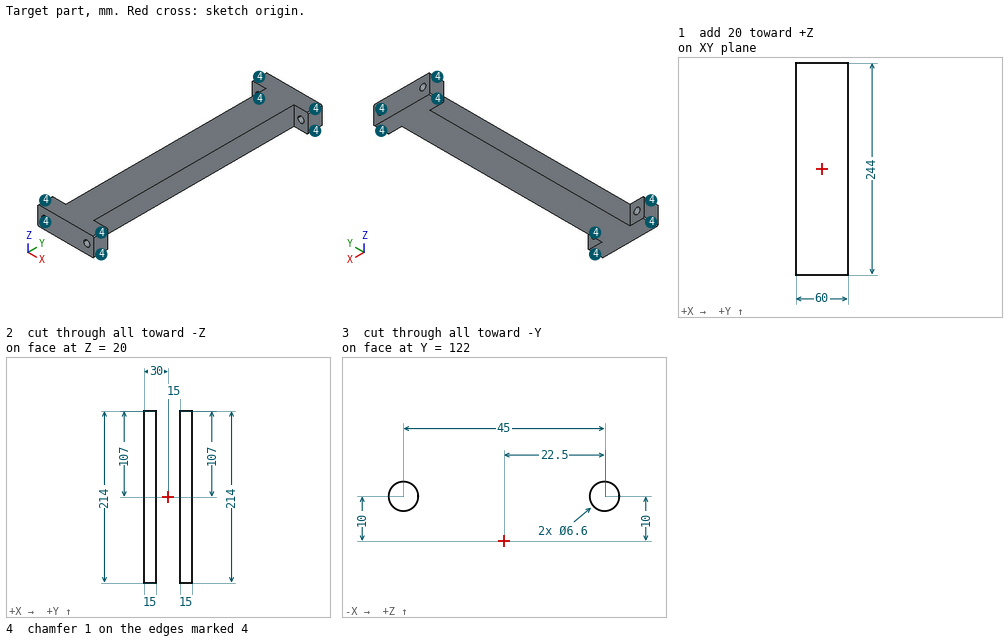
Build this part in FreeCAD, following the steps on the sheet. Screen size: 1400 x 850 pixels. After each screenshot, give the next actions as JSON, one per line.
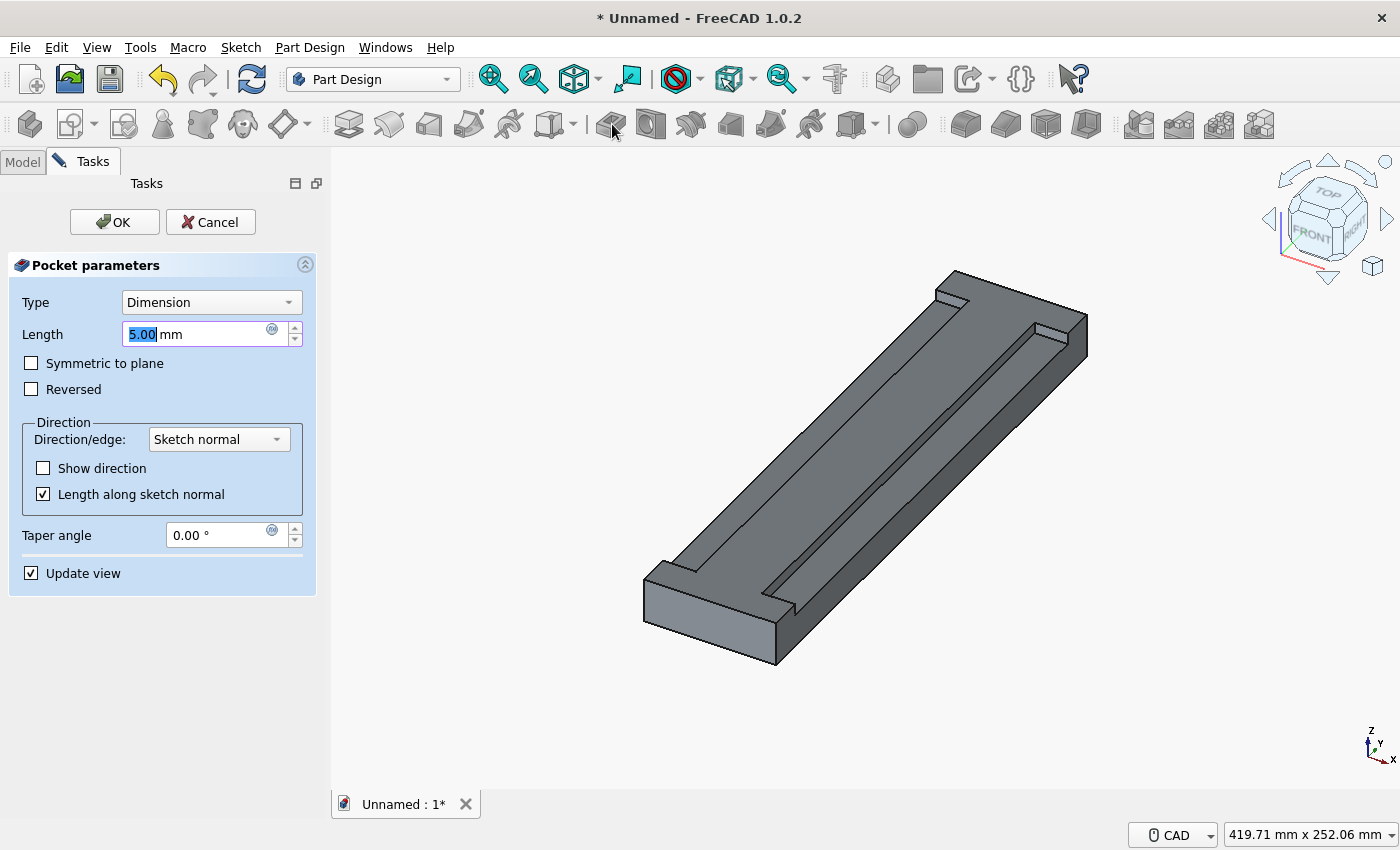
{"action": "left_click", "coordinate": [212, 302]}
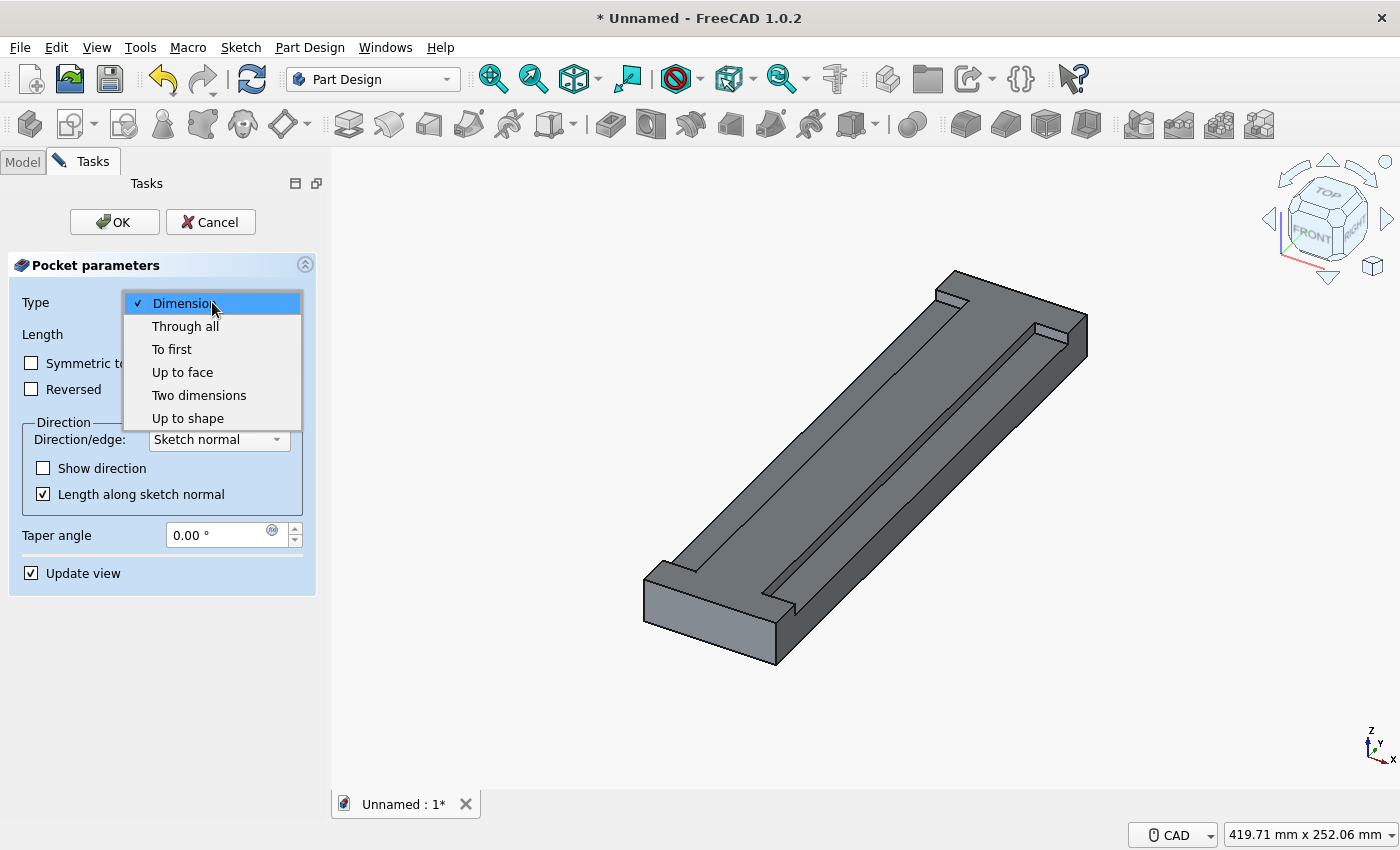
{"action": "left_click", "coordinate": [212, 326]}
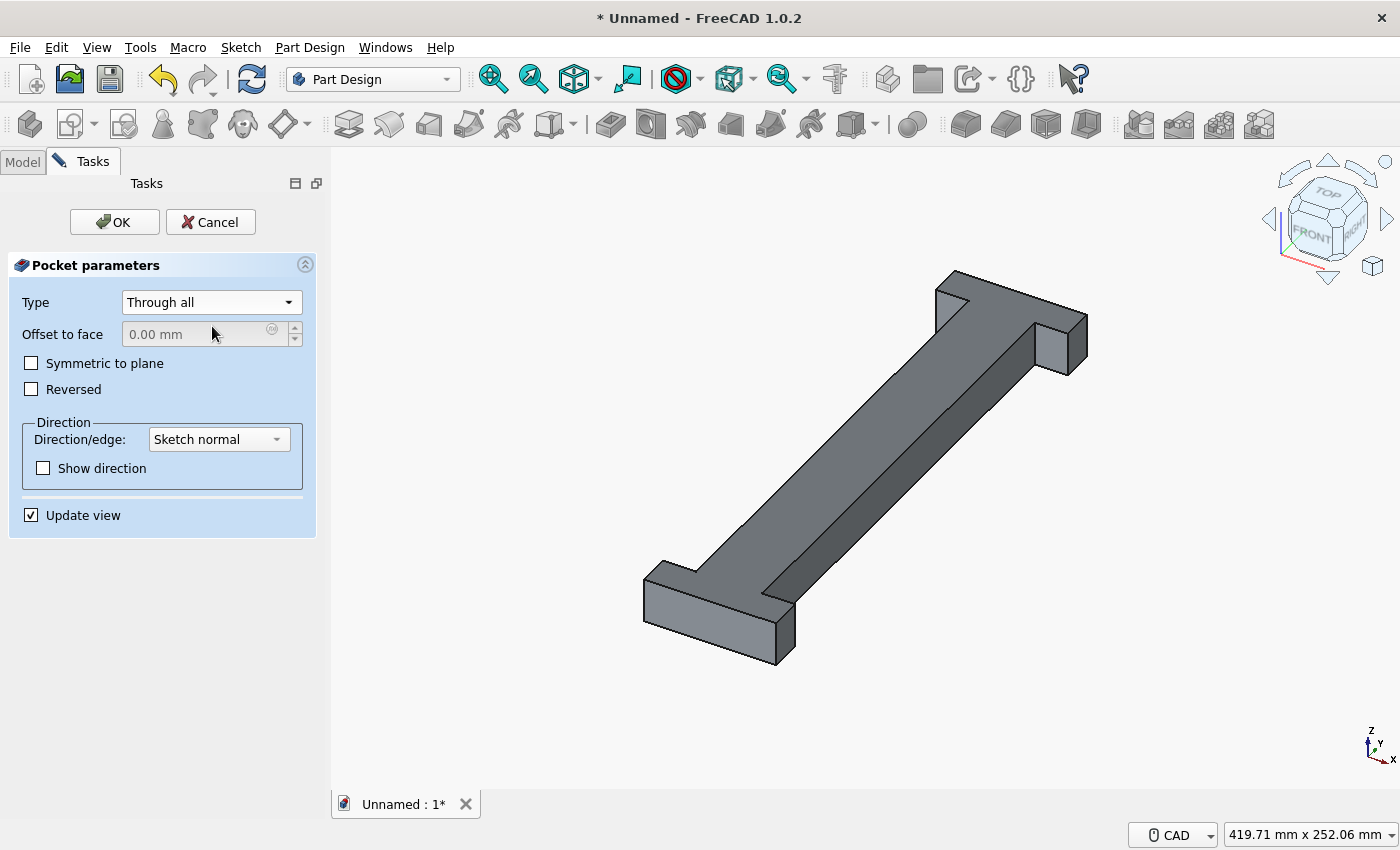
{"action": "left_click", "coordinate": [115, 222]}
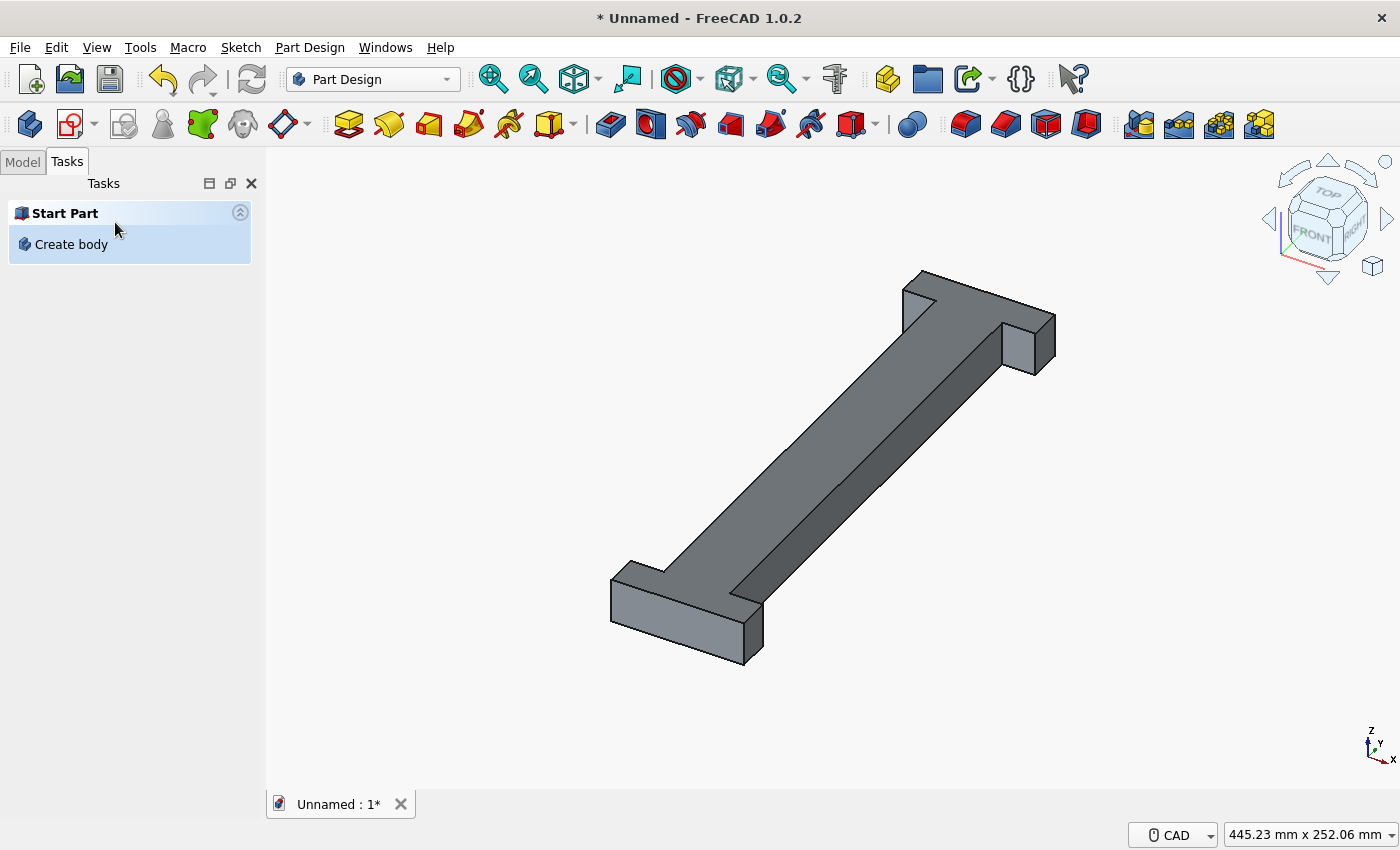
{"action": "key", "text": "4"}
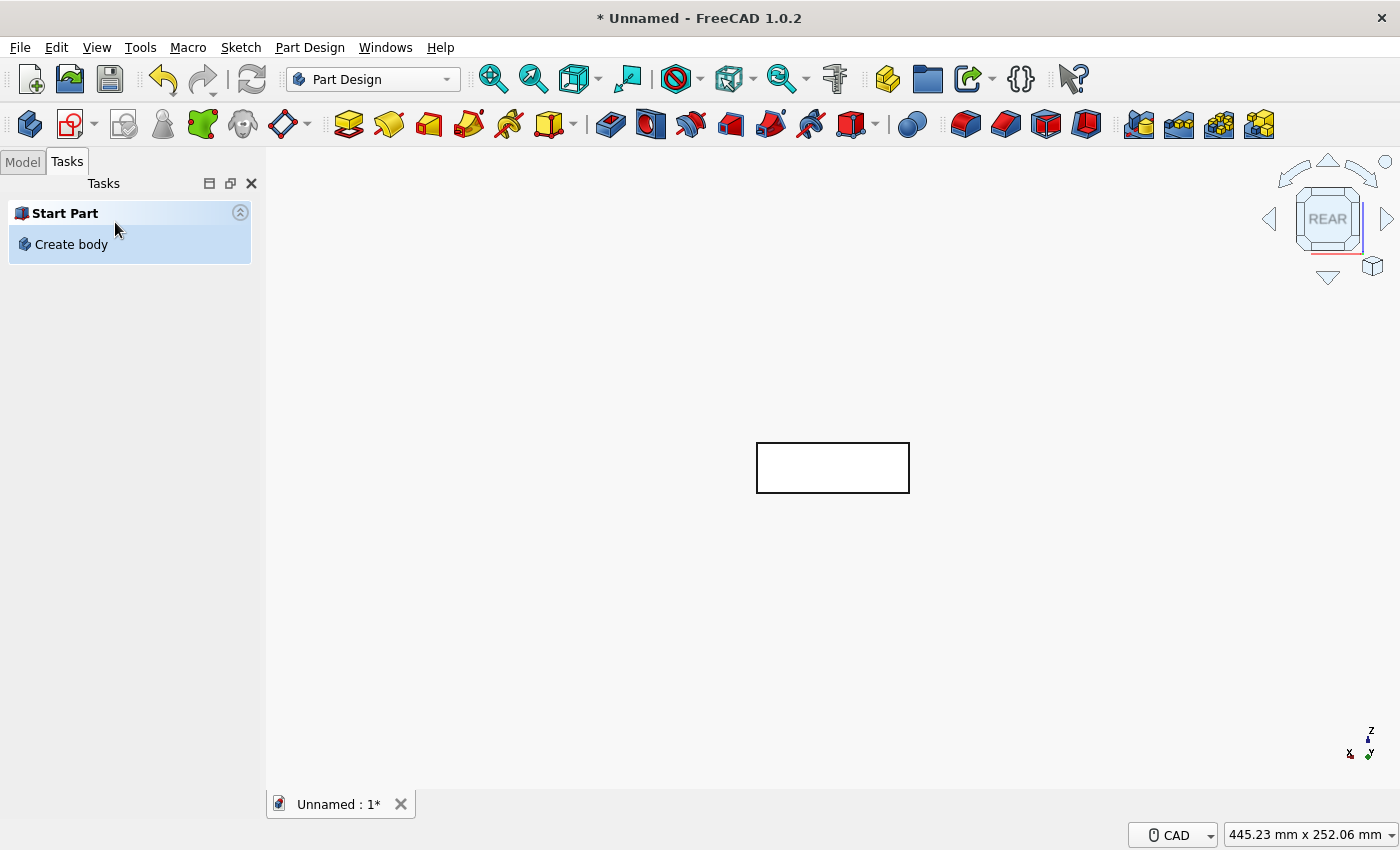
{"action": "left_click", "coordinate": [494, 80]}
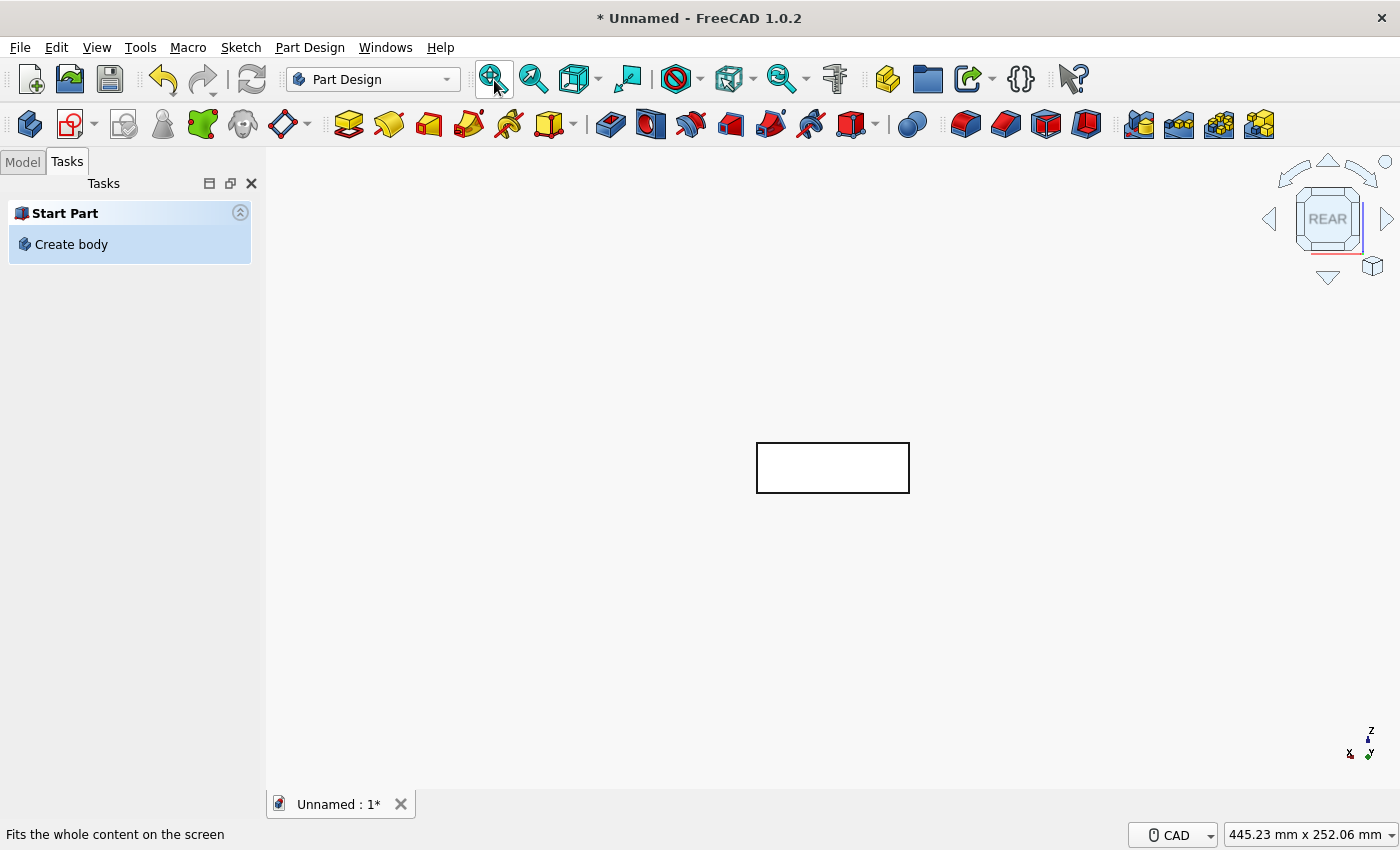
{"action": "left_click", "coordinate": [789, 467]}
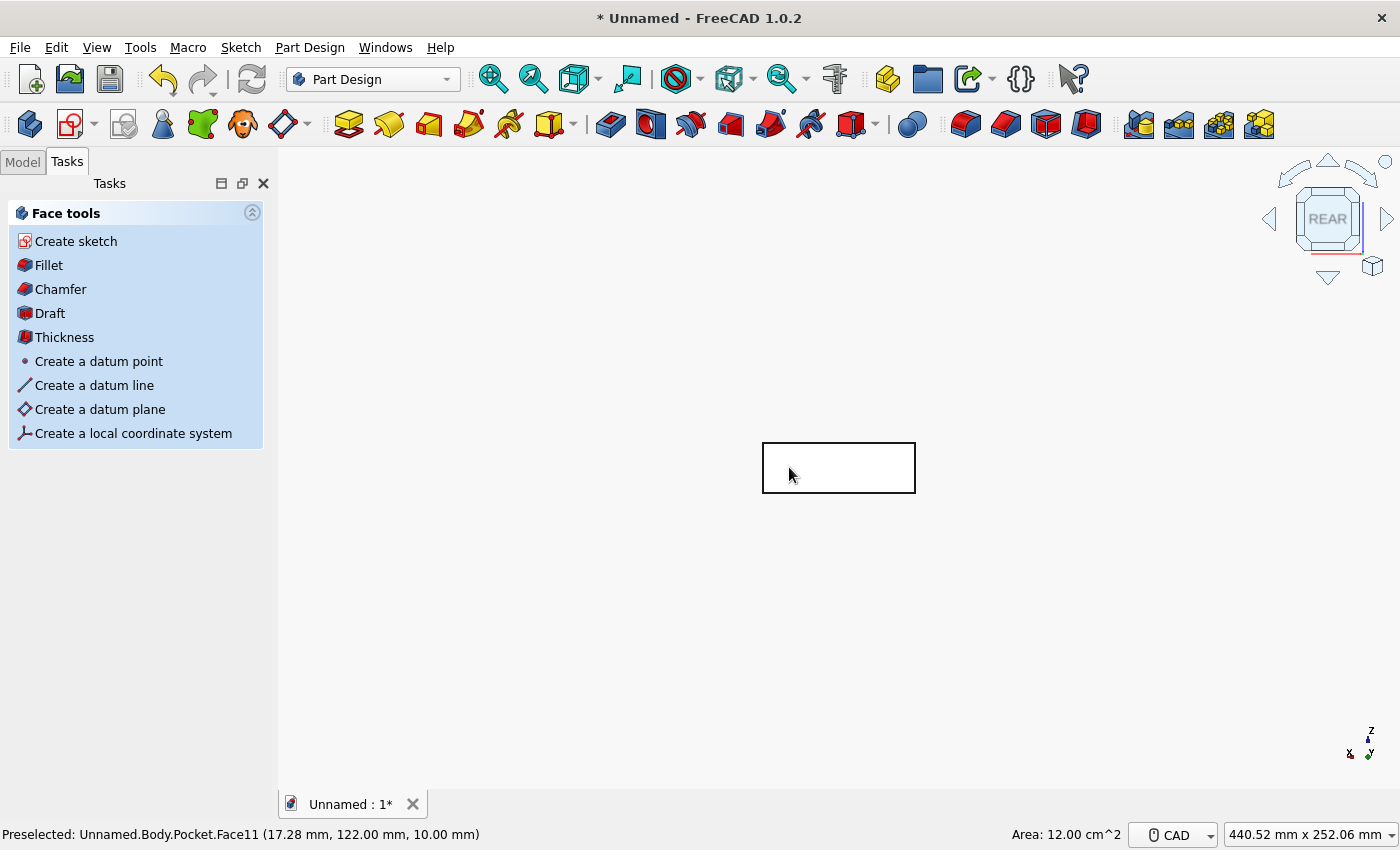
{"action": "left_click", "coordinate": [70, 124]}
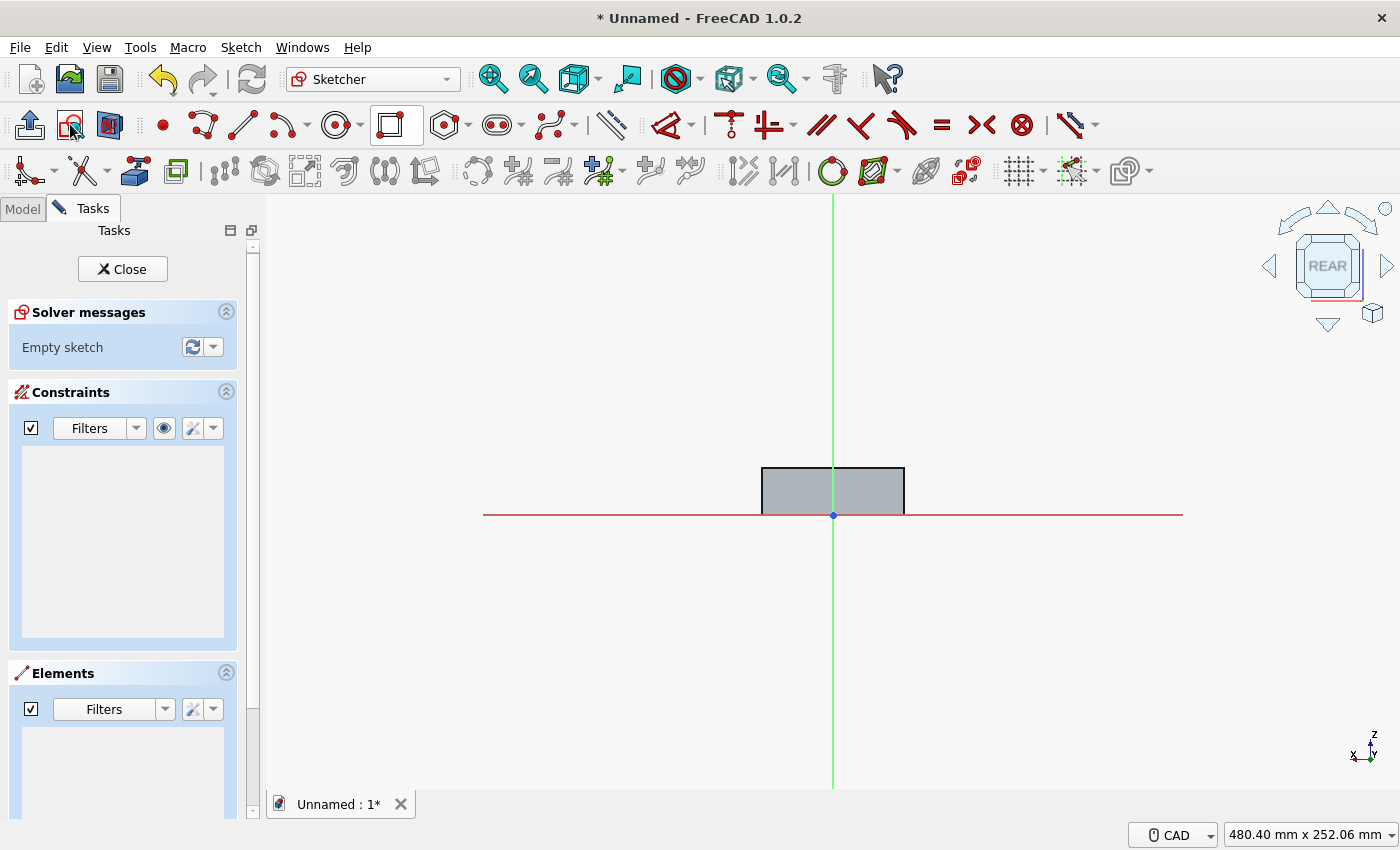
{"action": "scroll", "coordinate": [850, 501], "scroll_direction": "up", "scroll_amount": 8}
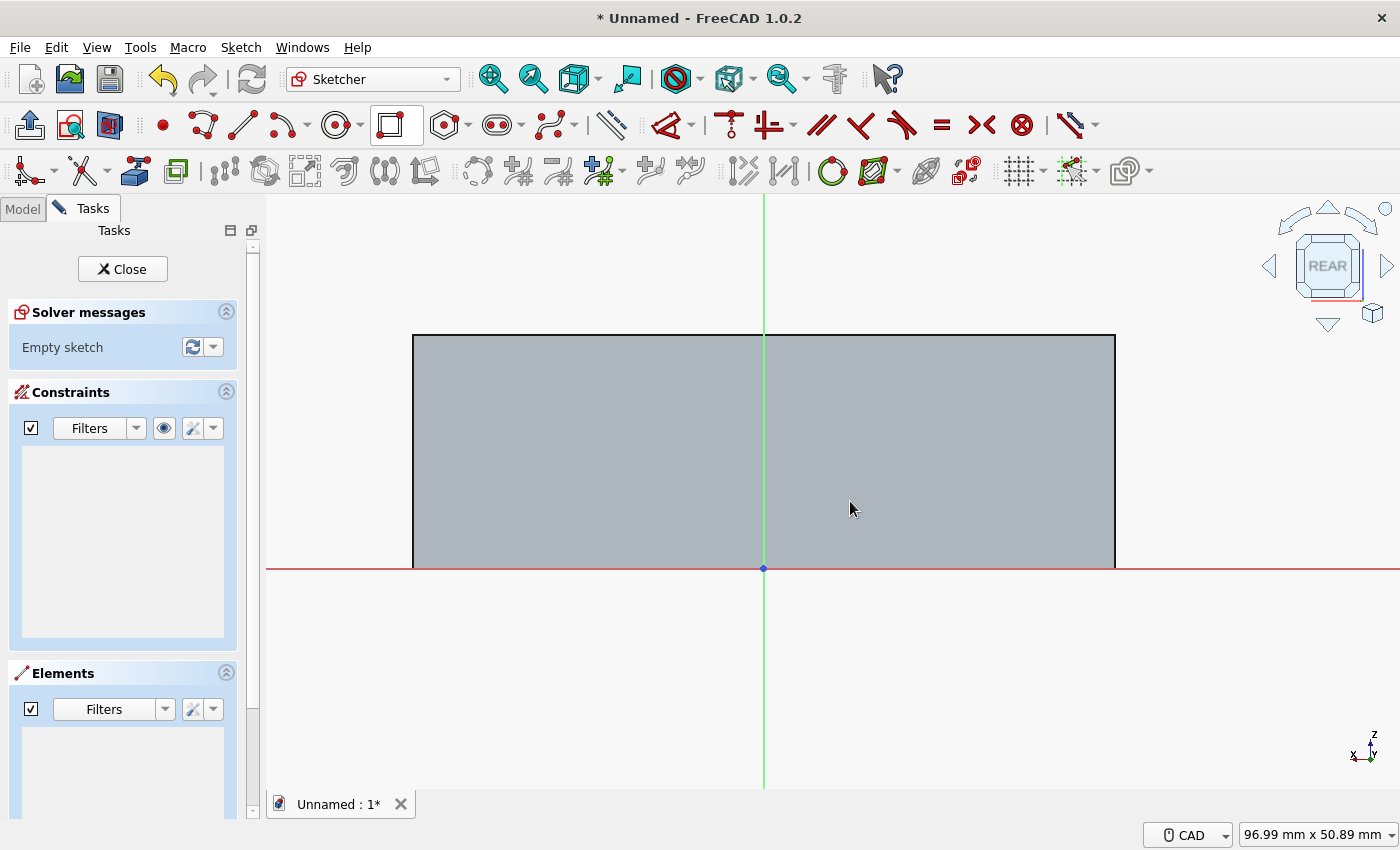
{"action": "left_click", "coordinate": [336, 126]}